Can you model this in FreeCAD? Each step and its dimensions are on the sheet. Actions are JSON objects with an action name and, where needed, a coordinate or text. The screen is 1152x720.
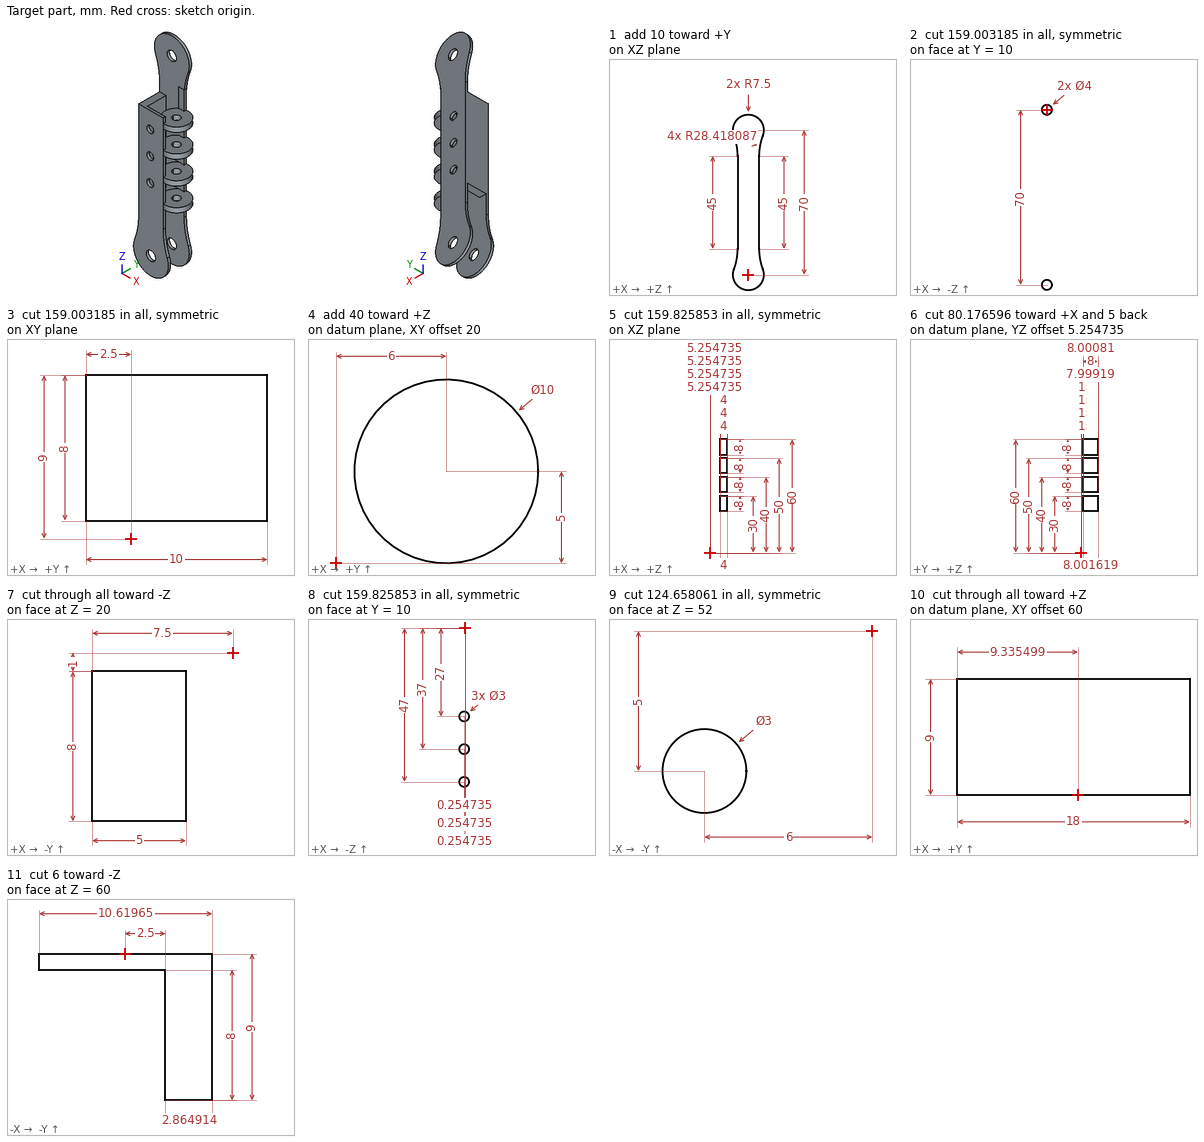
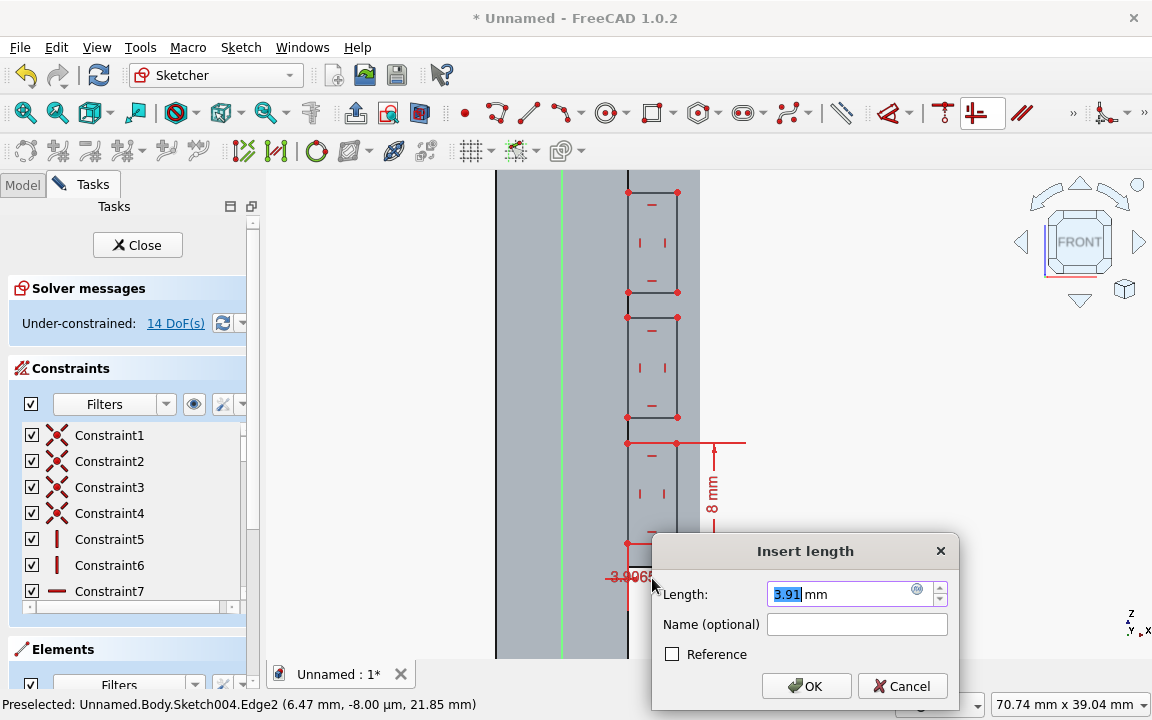
{"action": "type", "text": "4"}
{"action": "key", "text": "Return"}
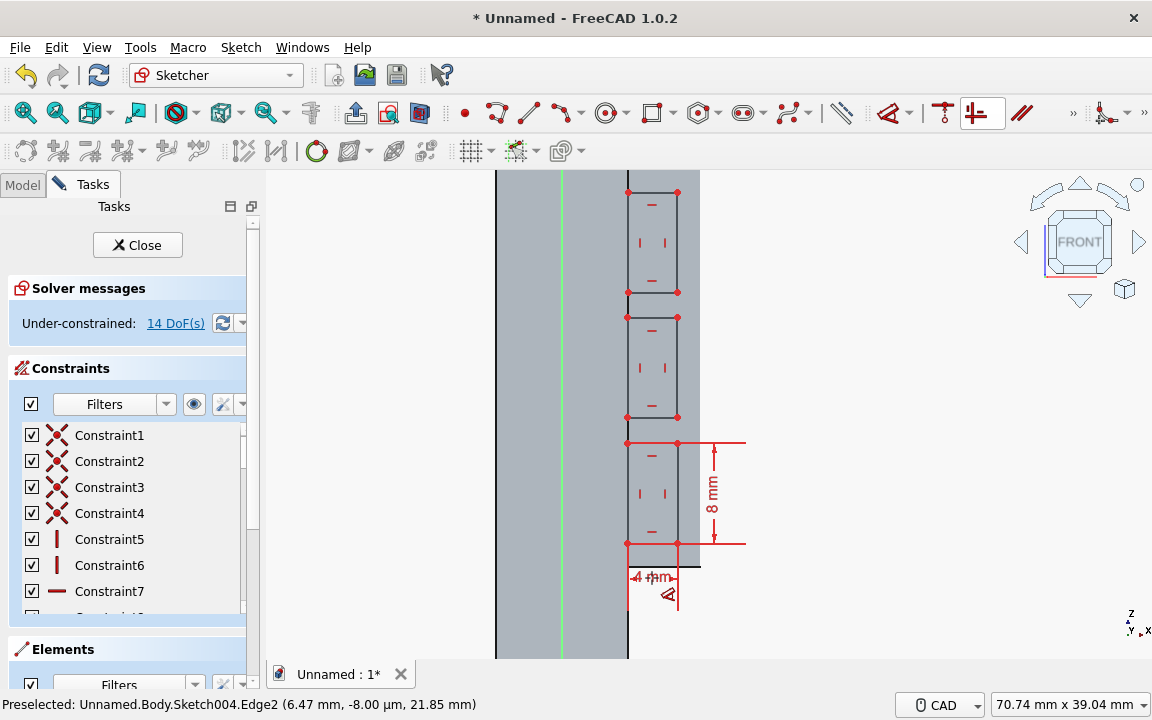
{"action": "left_click", "coordinate": [628, 348]}
{"action": "left_click", "coordinate": [662, 368]}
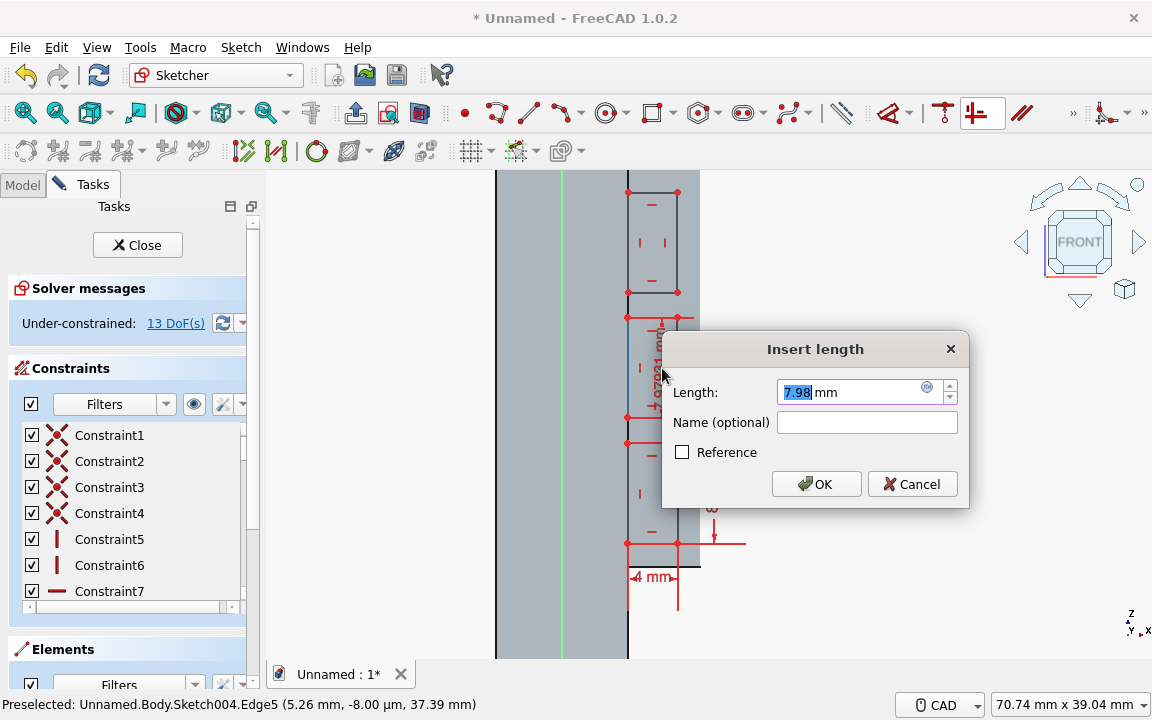
{"action": "type", "text": "8"}
{"action": "key", "text": "Return"}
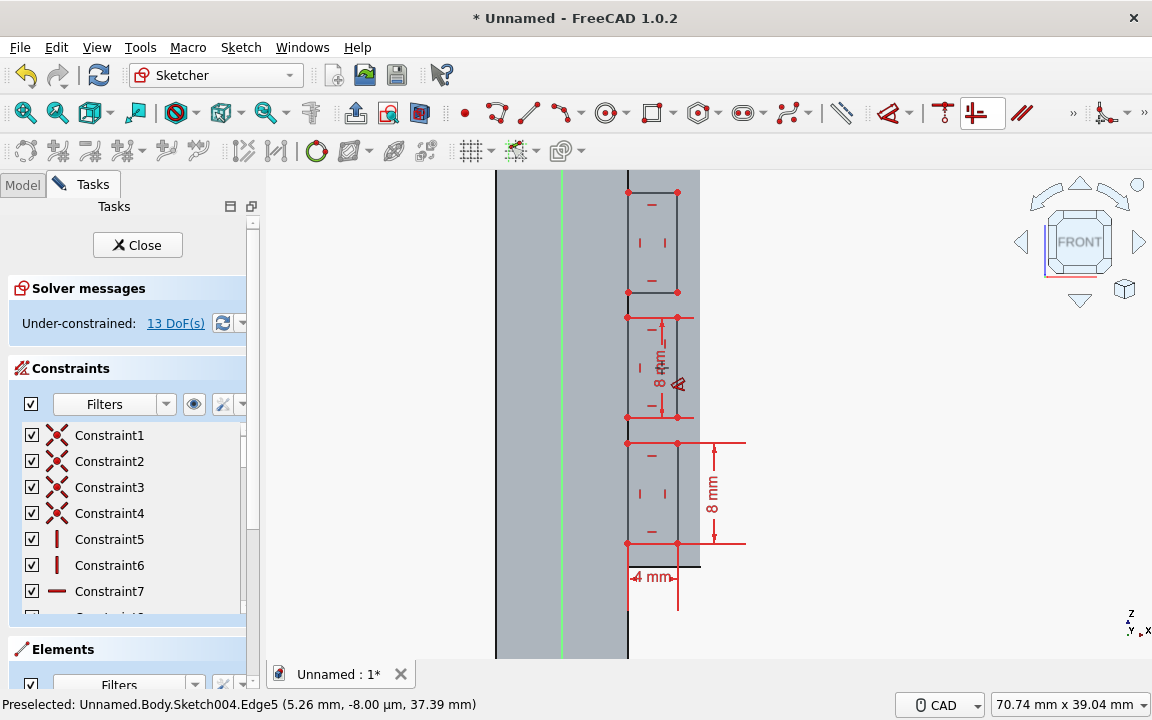
{"action": "left_click", "coordinate": [643, 418]}
{"action": "left_click", "coordinate": [641, 476]}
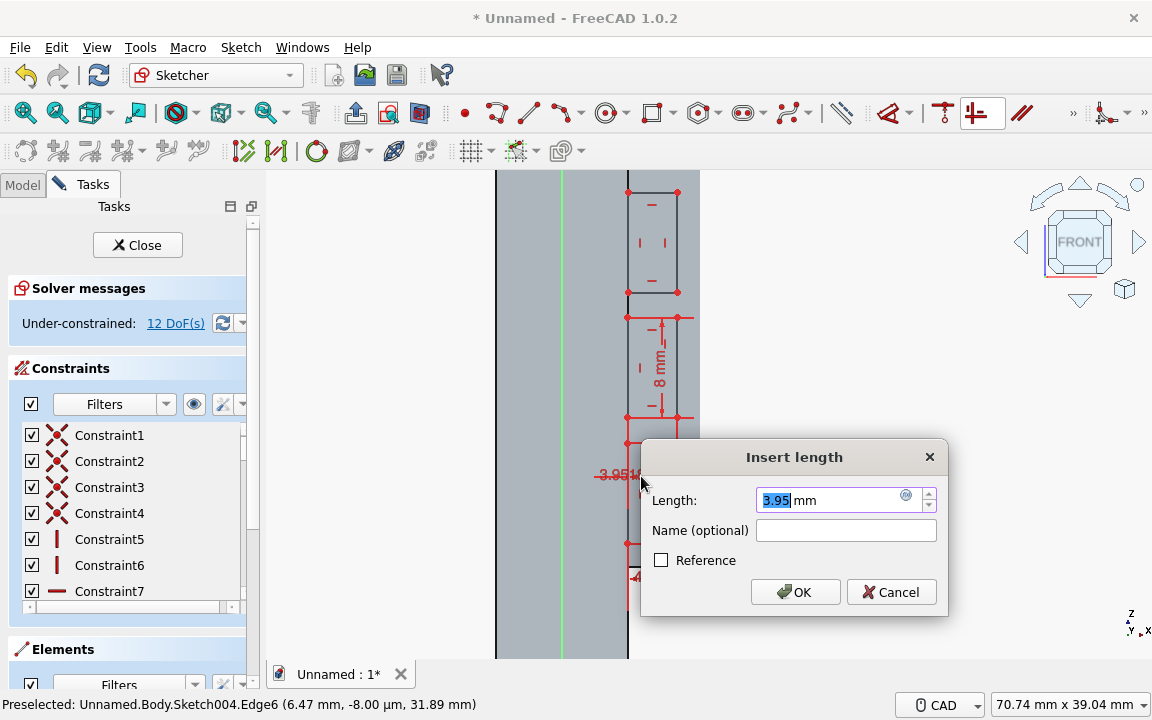
{"action": "type", "text": "4"}
{"action": "key", "text": "Return"}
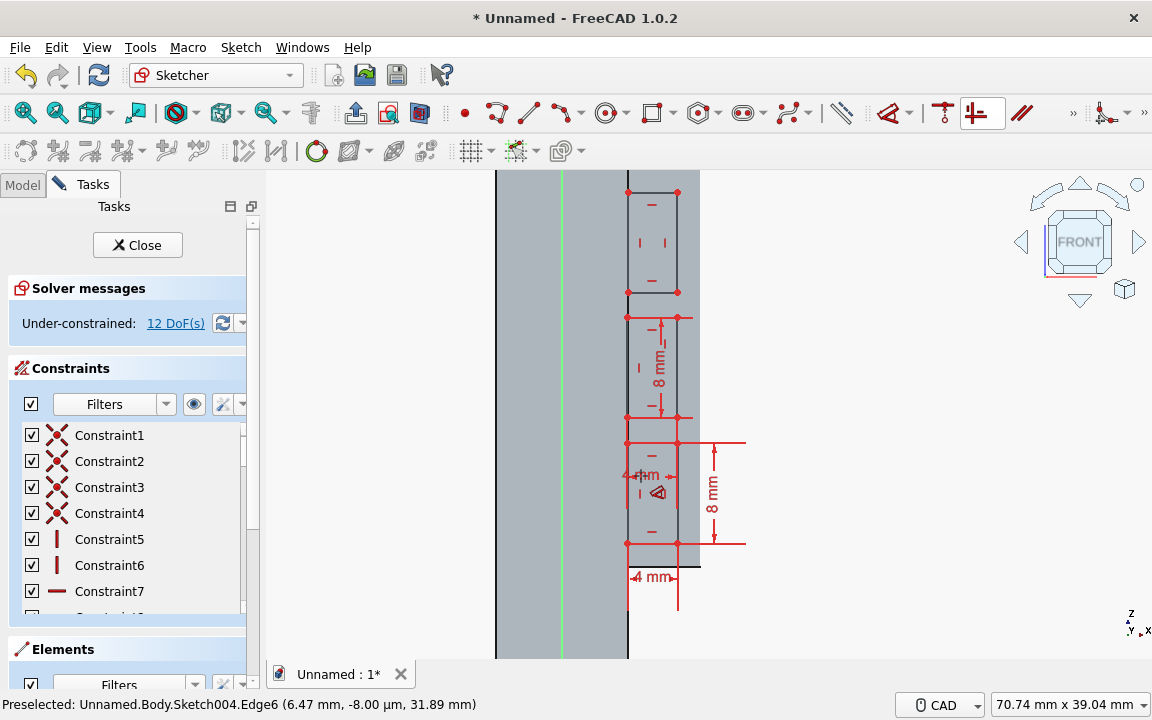
{"action": "left_click", "coordinate": [628, 223]}
{"action": "left_click", "coordinate": [662, 245]}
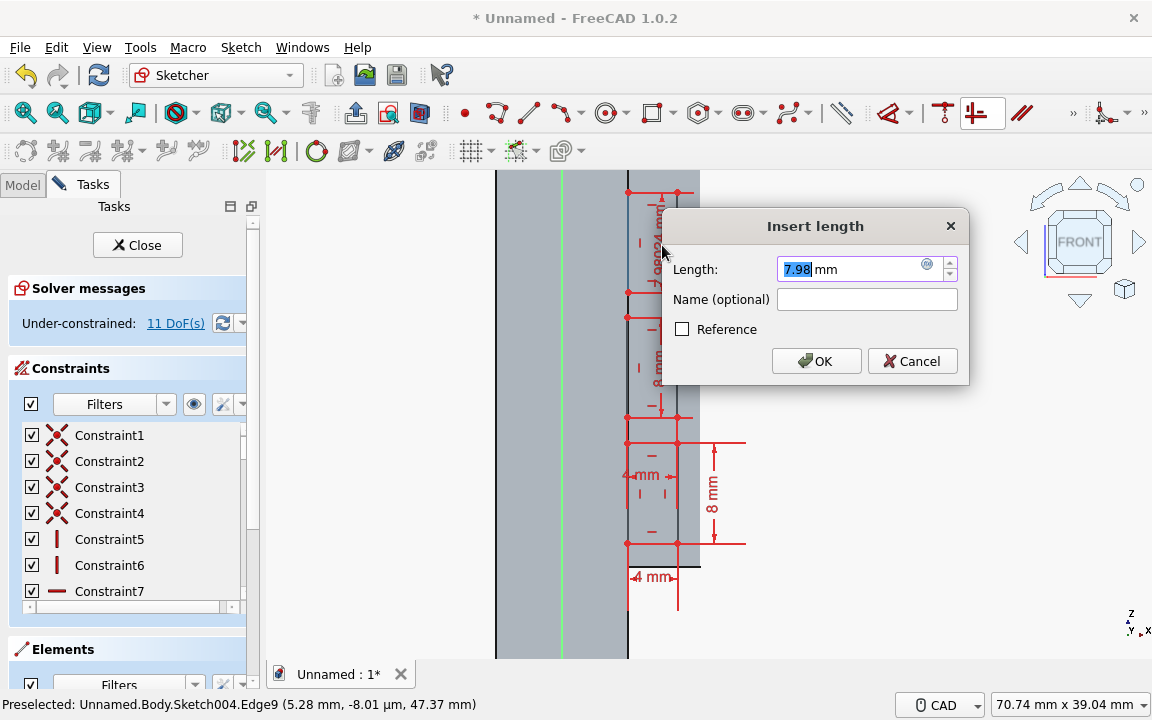
{"action": "type", "text": "8"}
{"action": "key", "text": "Return"}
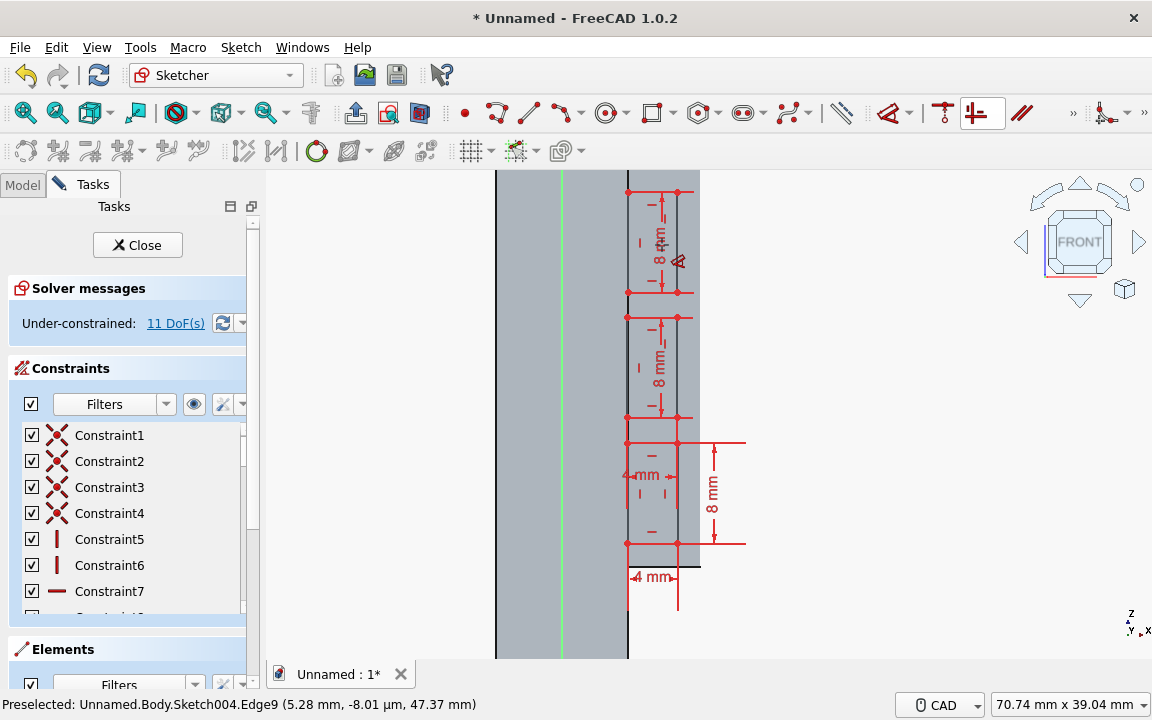
{"action": "left_click", "coordinate": [643, 293]}
{"action": "left_click", "coordinate": [653, 211]}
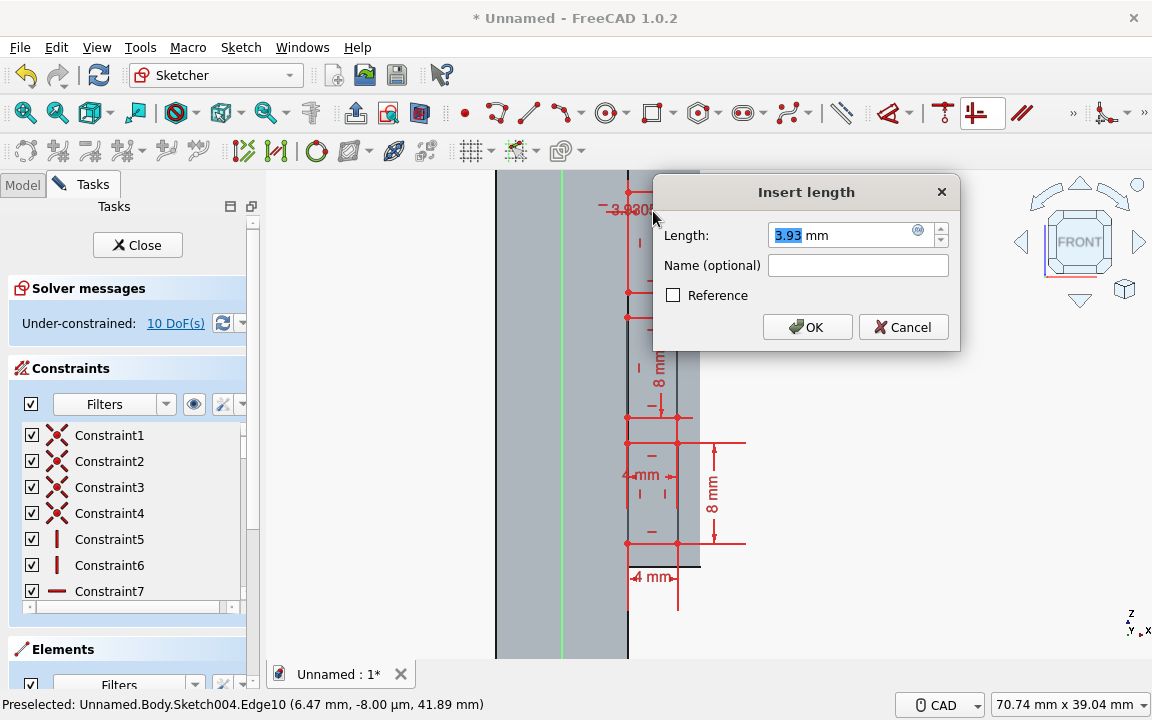
{"action": "type", "text": "4"}
{"action": "key", "text": "Return"}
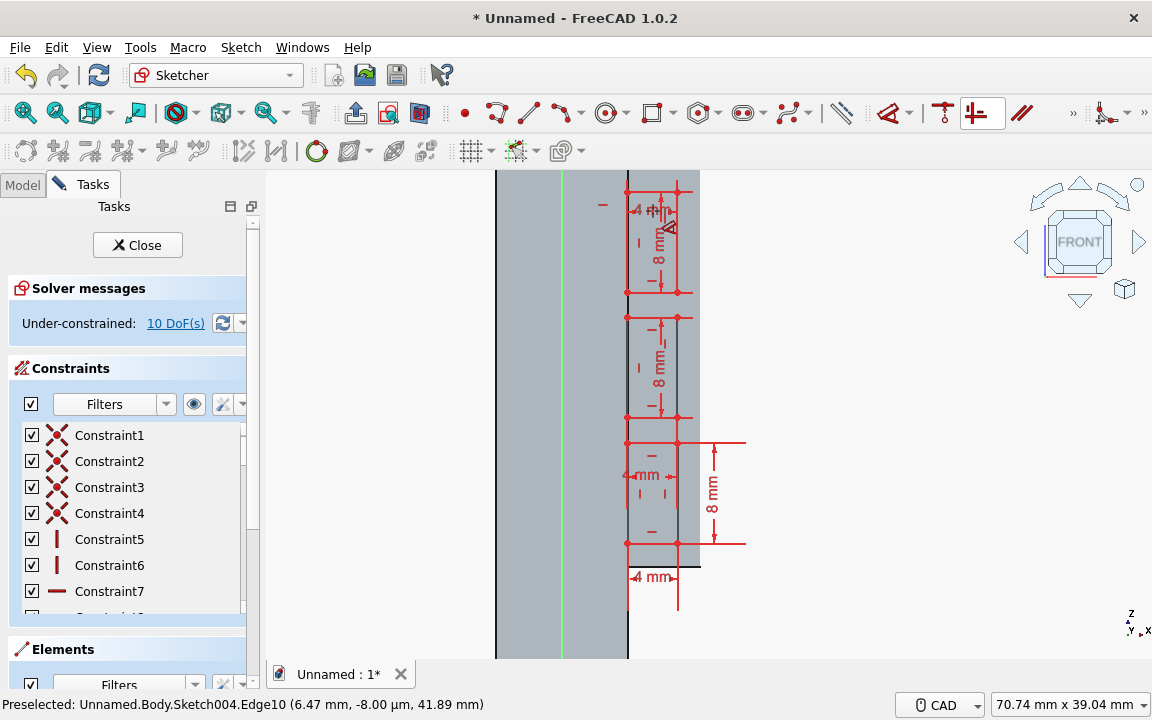
{"action": "scroll", "coordinate": [657, 392], "scroll_direction": "down", "scroll_amount": 4}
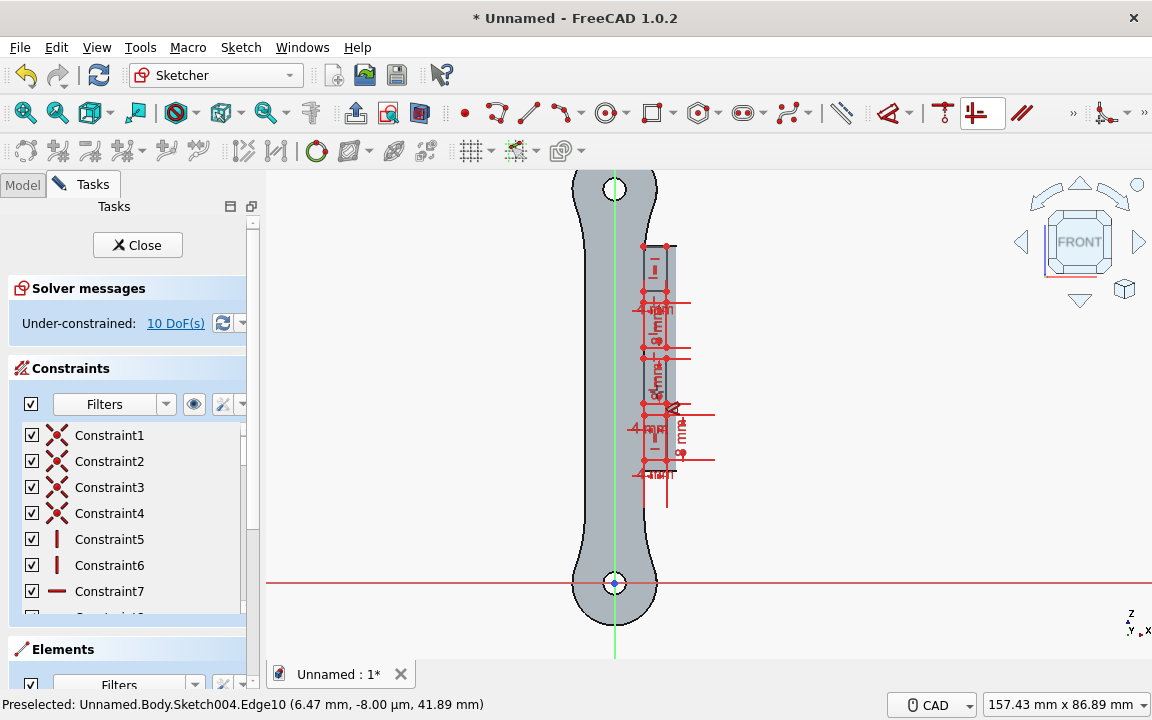
{"action": "left_click", "coordinate": [644, 260]}
{"action": "left_click", "coordinate": [702, 269]}